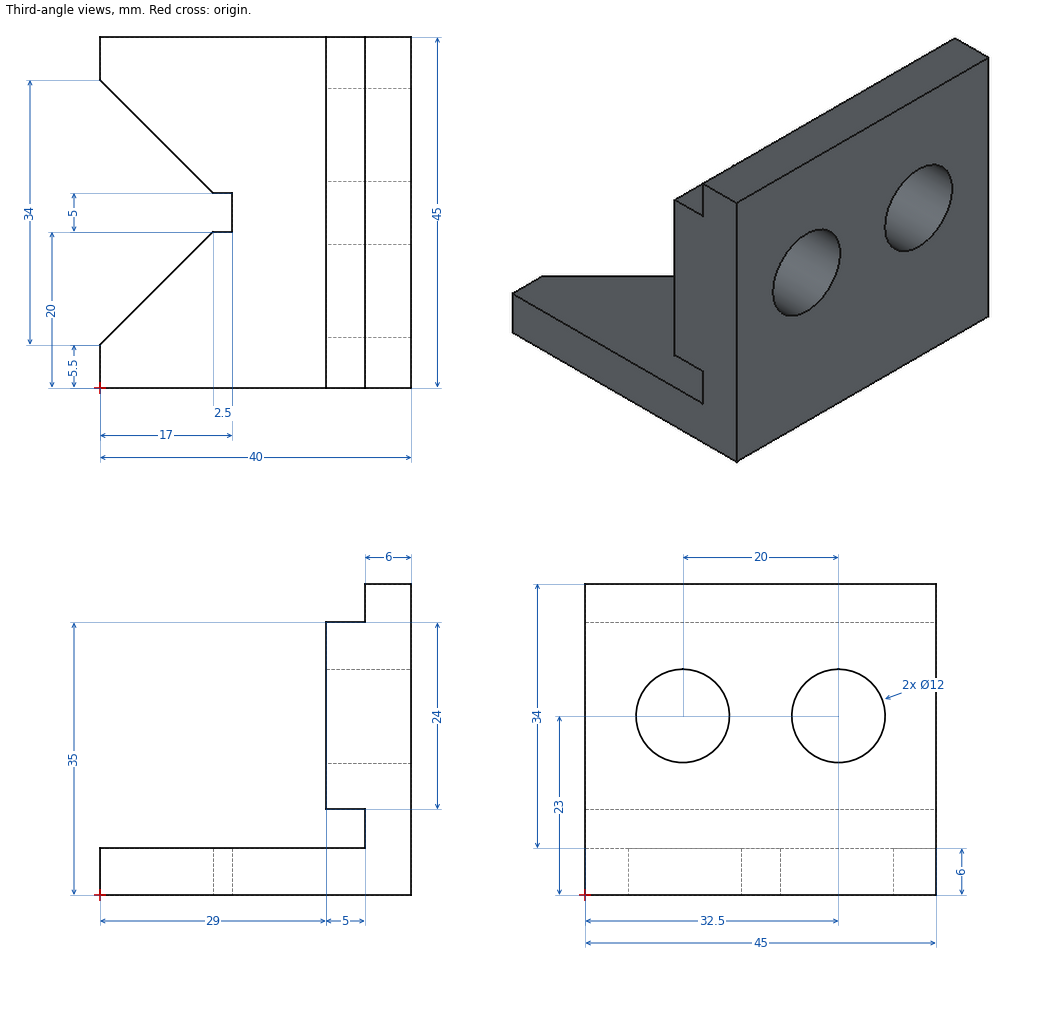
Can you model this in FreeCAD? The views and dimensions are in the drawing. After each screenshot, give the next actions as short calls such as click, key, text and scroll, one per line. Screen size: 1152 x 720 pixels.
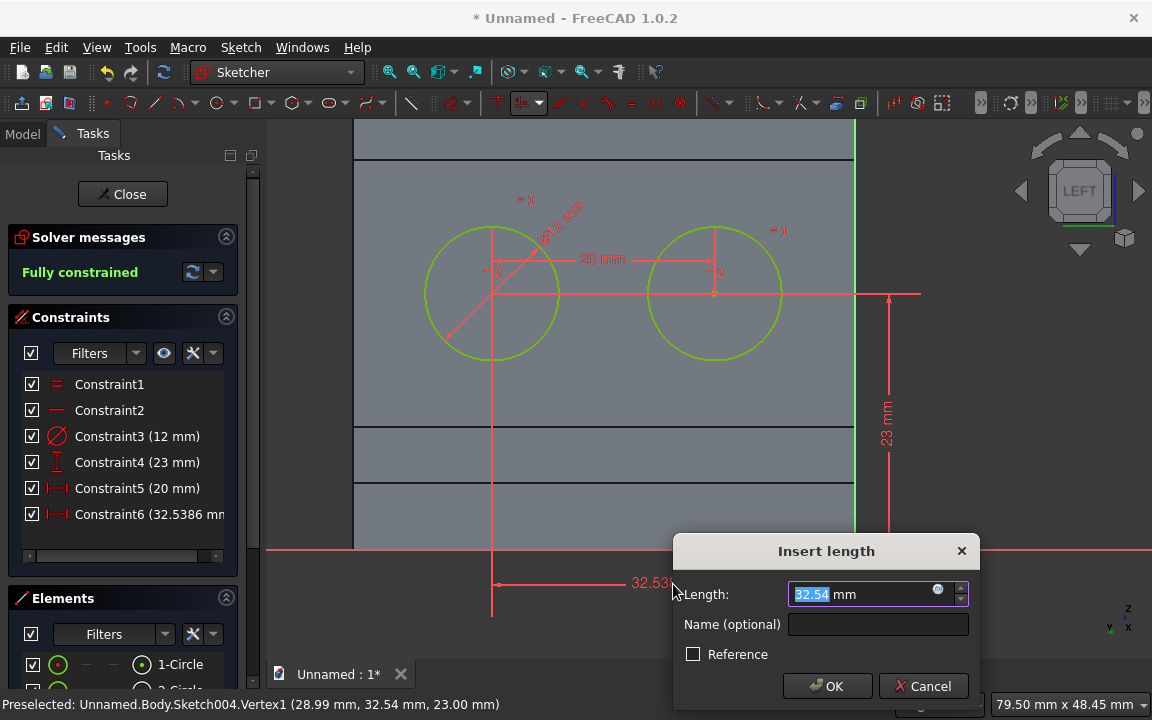
text(32.5)
key(Return)
key(Escape)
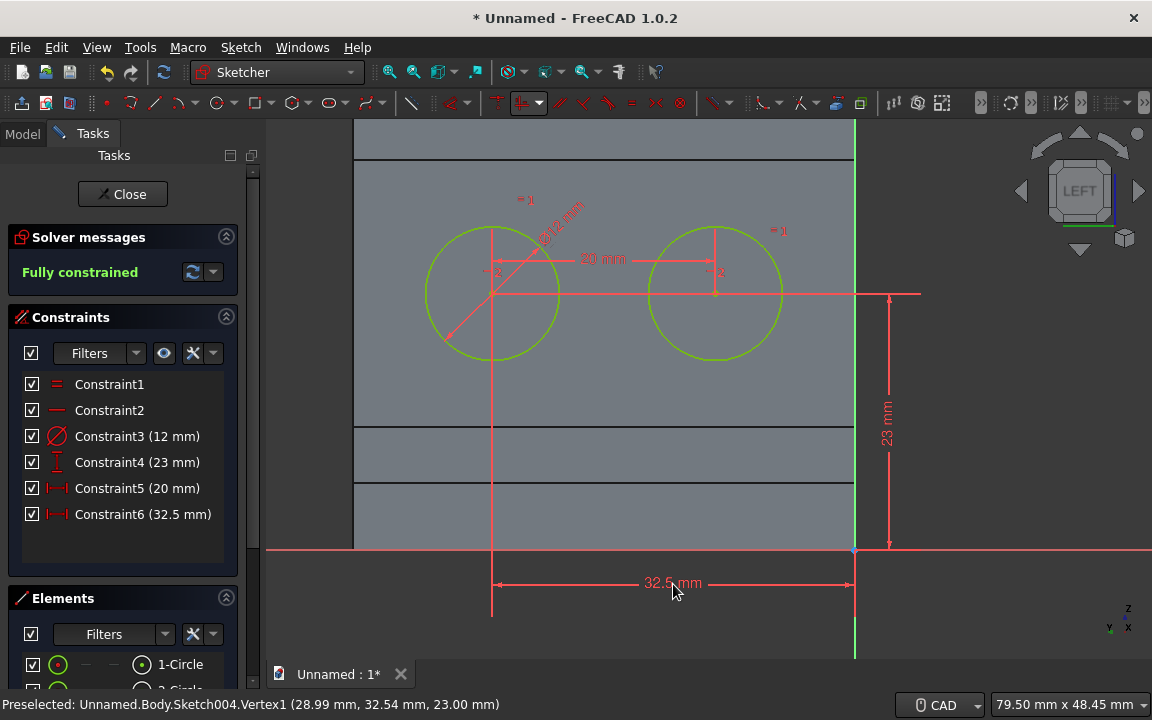
click(123, 194)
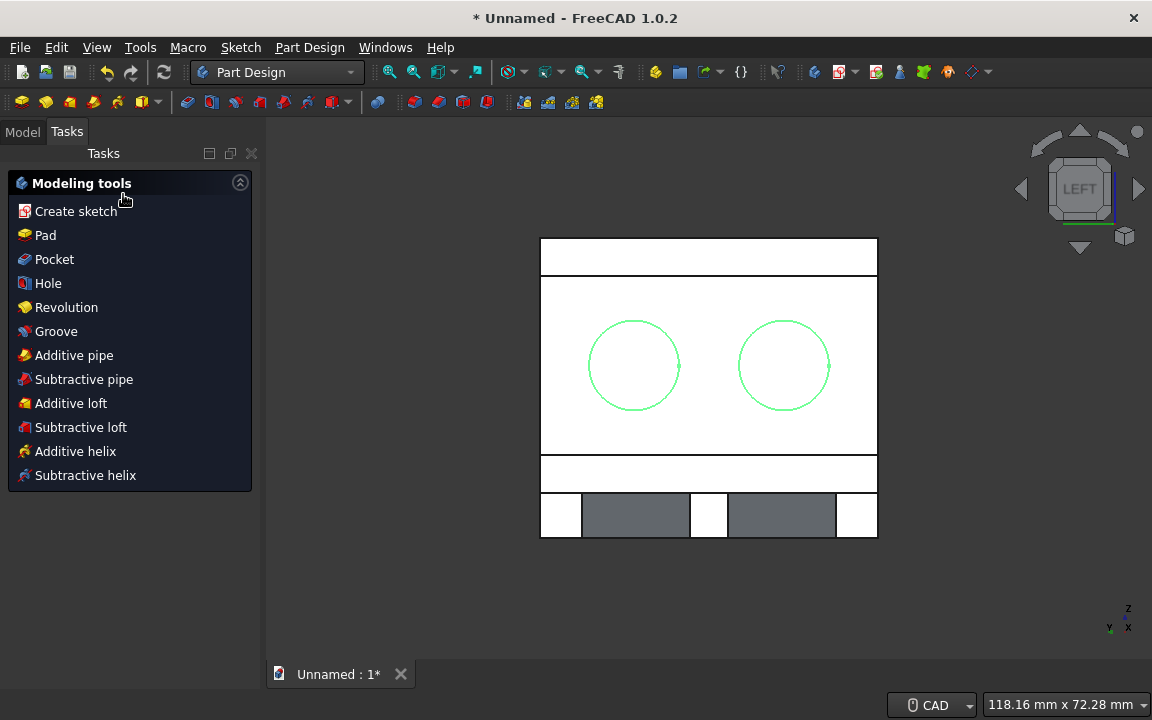
click(188, 102)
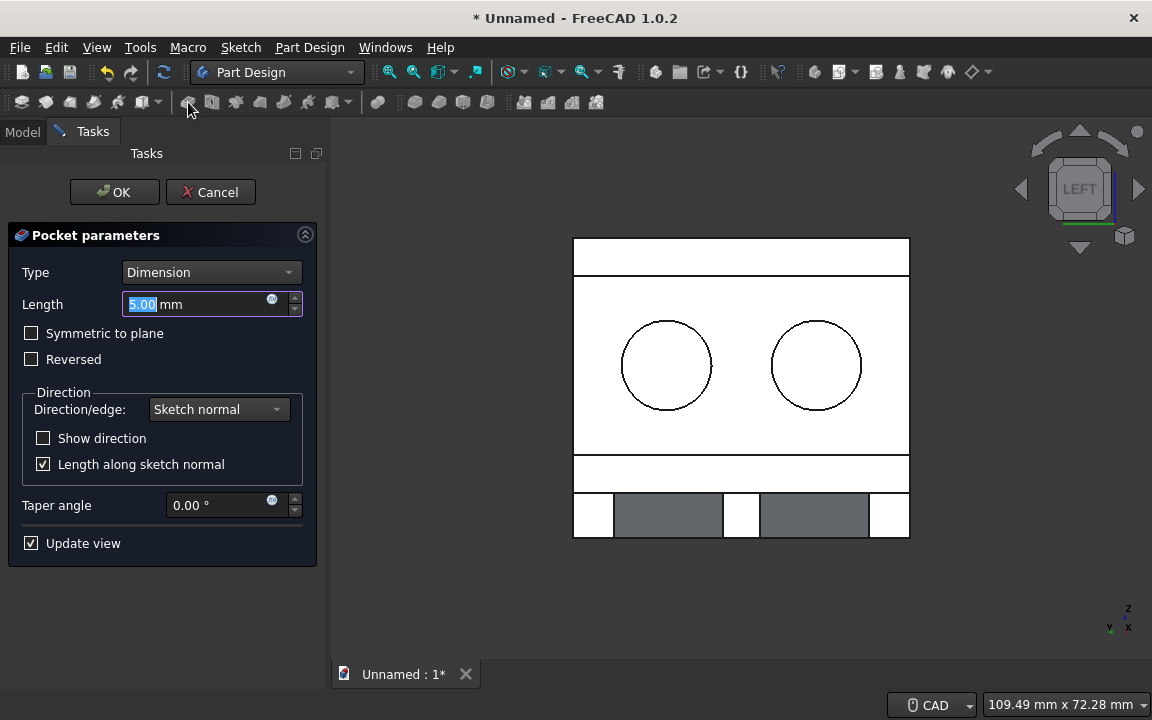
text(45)
key(Tab)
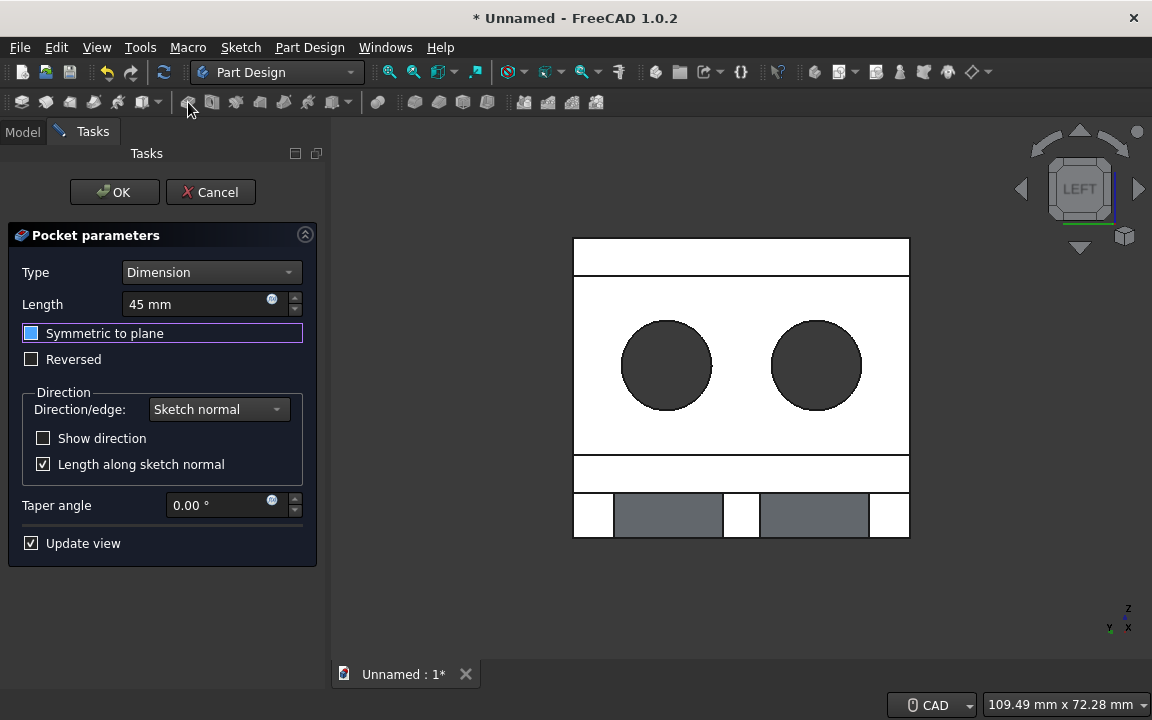
click(115, 192)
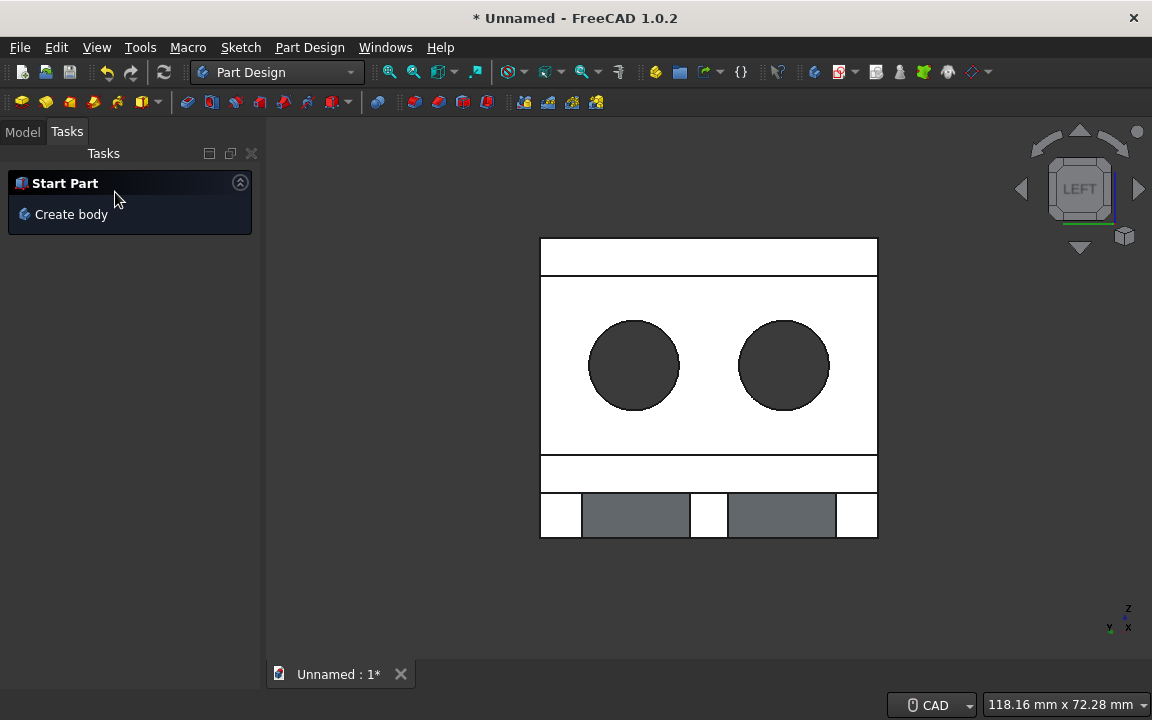
key(0)